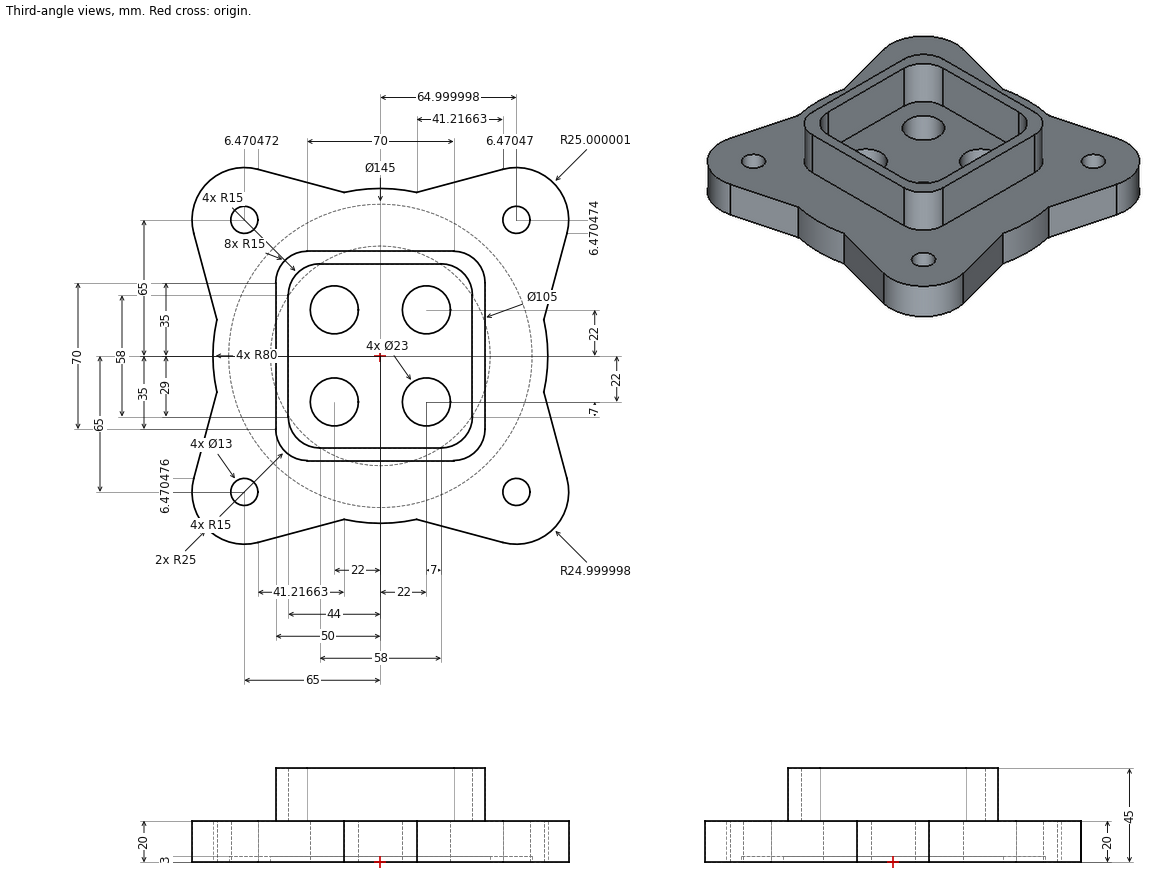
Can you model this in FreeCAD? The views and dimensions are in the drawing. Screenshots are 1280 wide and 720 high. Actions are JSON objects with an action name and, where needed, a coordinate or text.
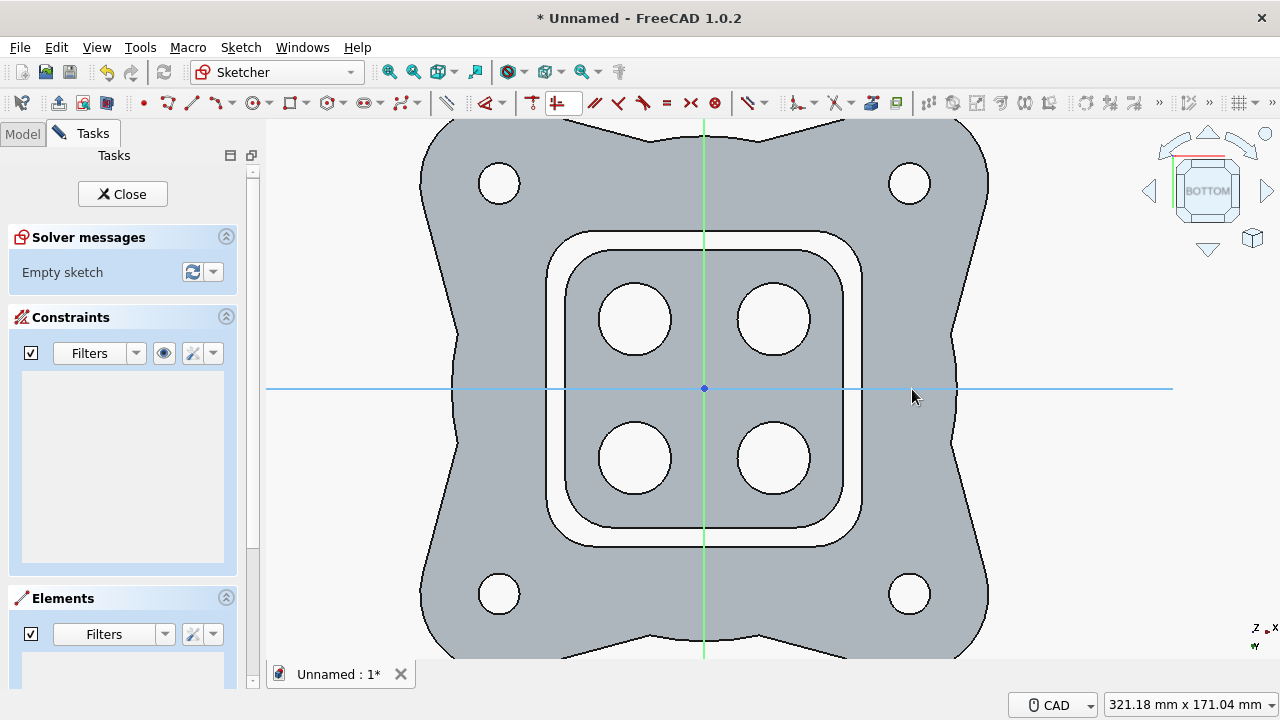
{"action": "key", "text": "g l"}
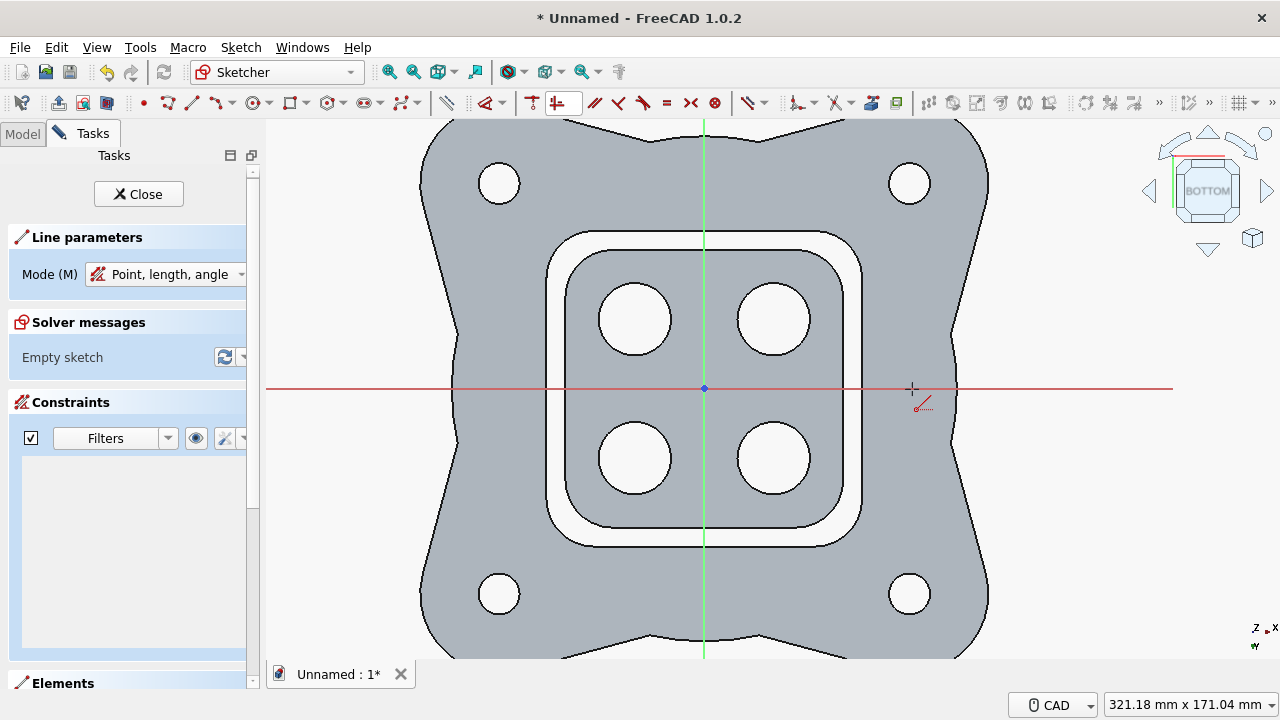
{"action": "left_click", "coordinate": [546, 499]}
{"action": "left_click", "coordinate": [546, 278]}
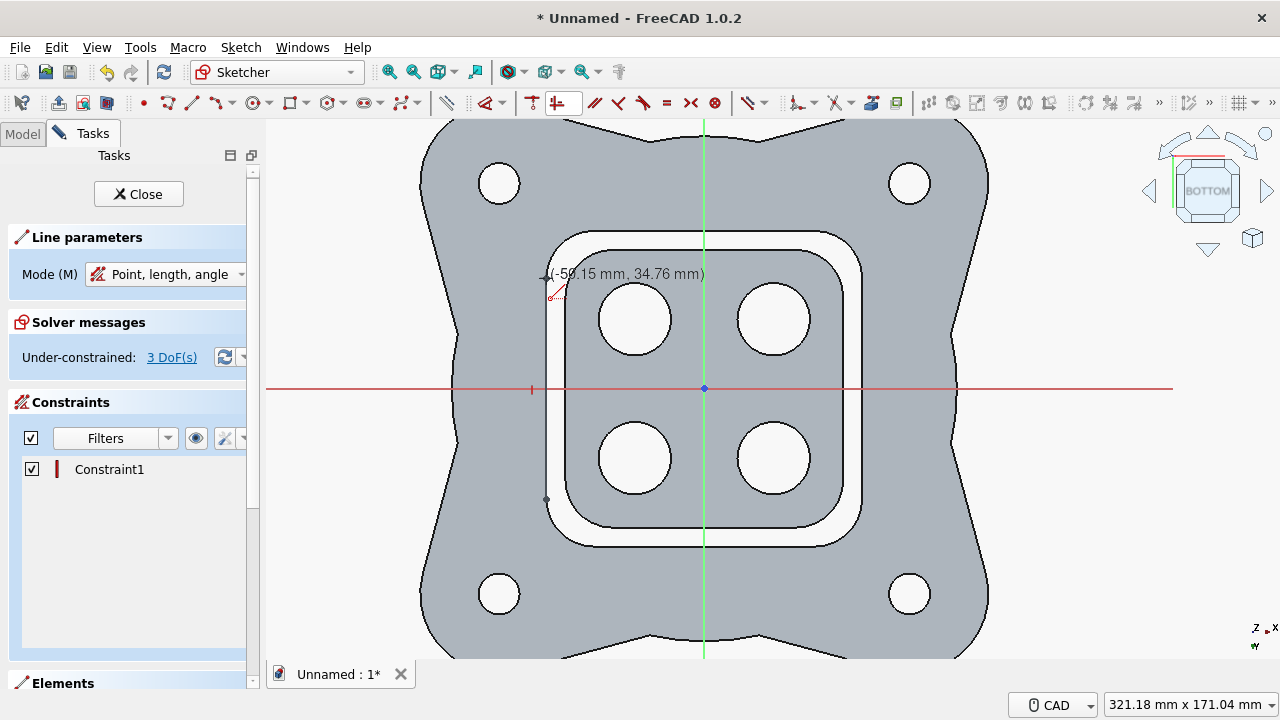
{"action": "left_click", "coordinate": [594, 231]}
{"action": "left_click", "coordinate": [815, 231]}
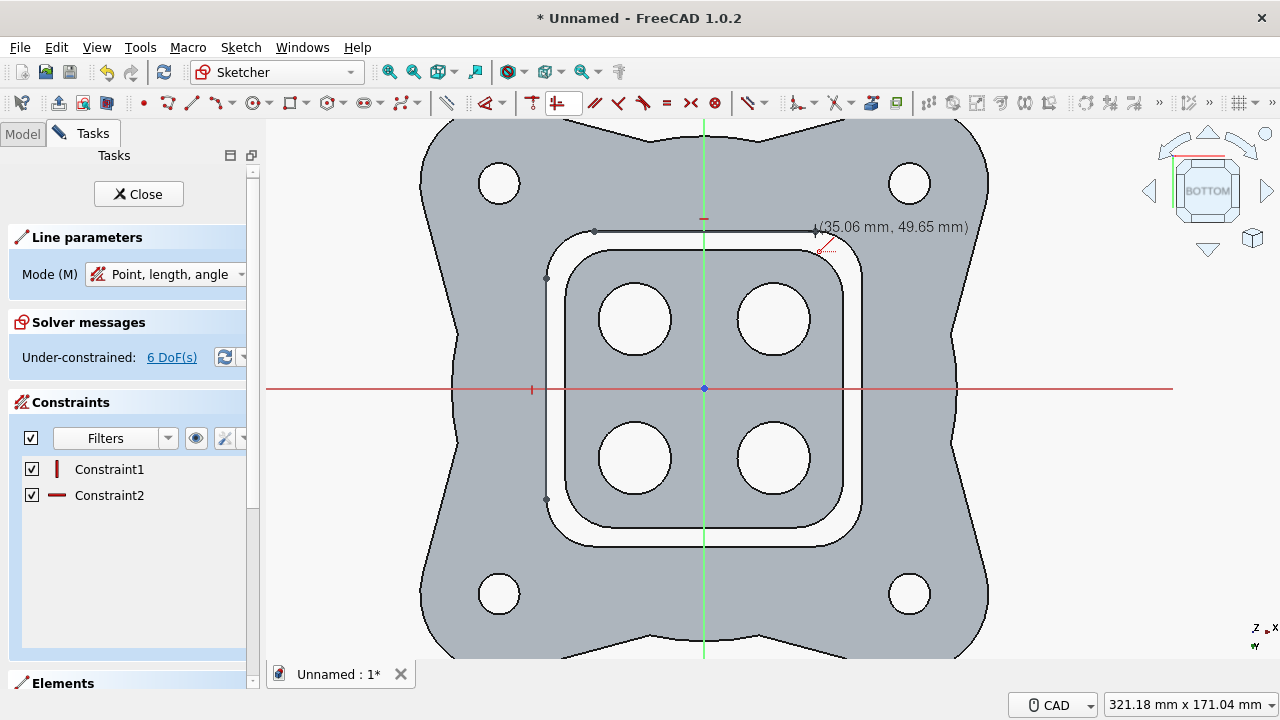
{"action": "left_click", "coordinate": [862, 278]}
{"action": "left_click", "coordinate": [862, 499]}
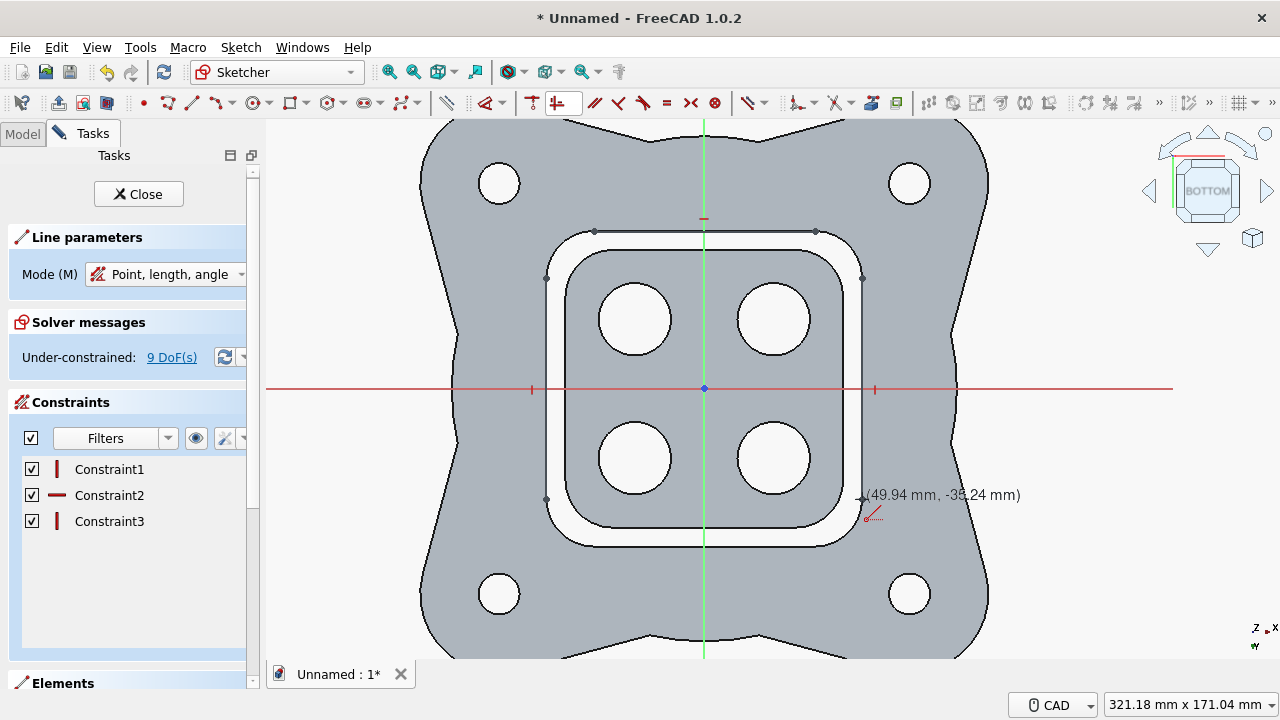
{"action": "left_click", "coordinate": [815, 547]}
{"action": "left_click", "coordinate": [594, 547]}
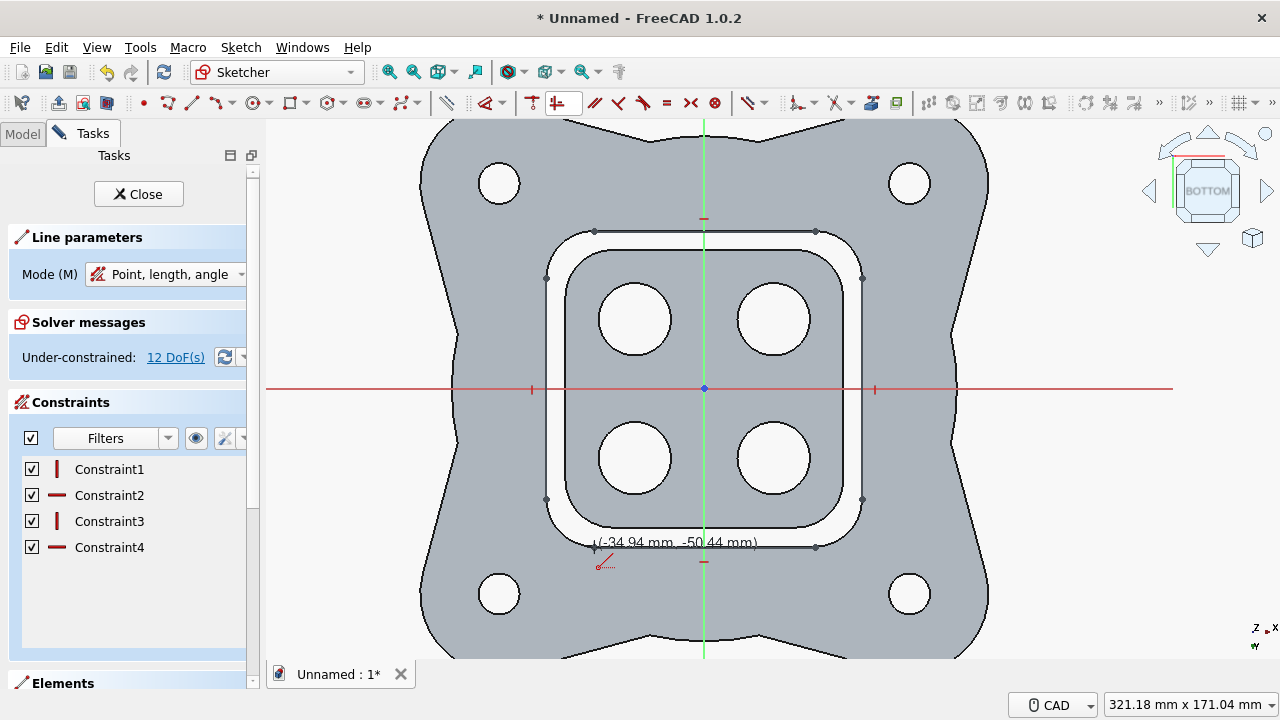
{"action": "key", "text": "g 3 a"}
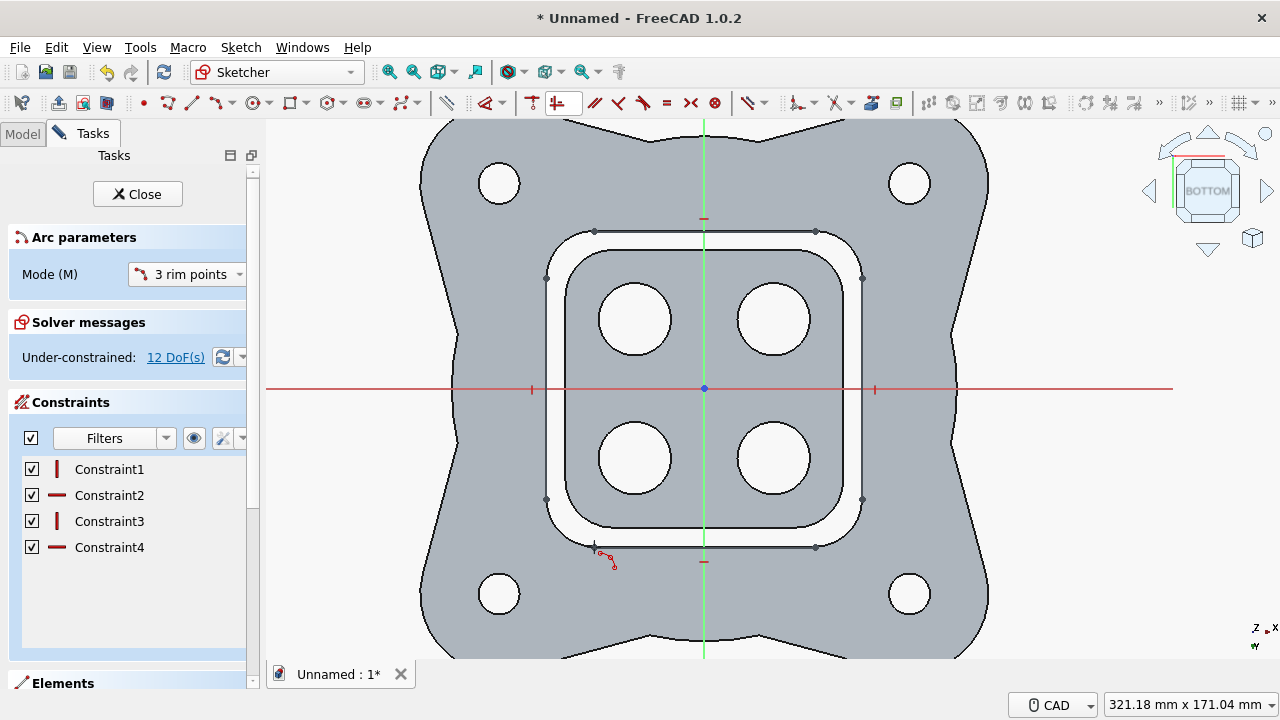
{"action": "left_click", "coordinate": [546, 279]}
{"action": "left_click", "coordinate": [594, 232]}
{"action": "left_click", "coordinate": [560, 245]}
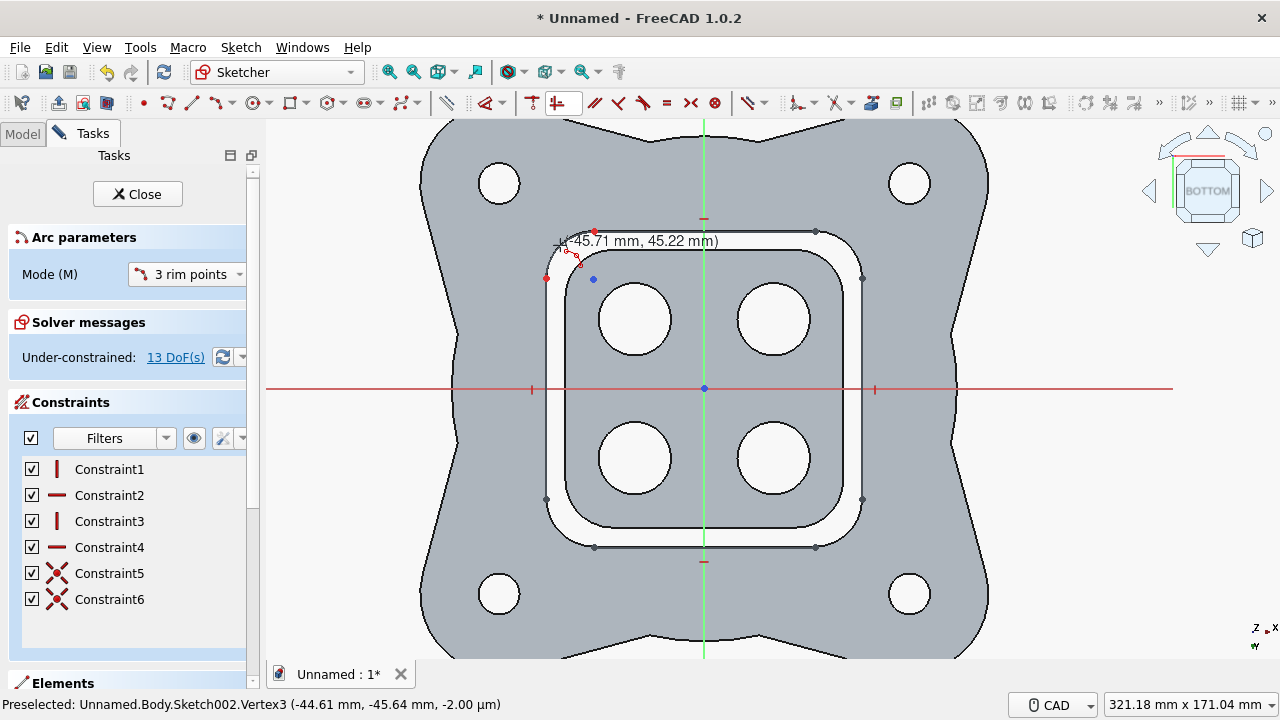
{"action": "left_click", "coordinate": [815, 232]}
{"action": "left_click", "coordinate": [862, 279]}
{"action": "left_click", "coordinate": [848, 245]}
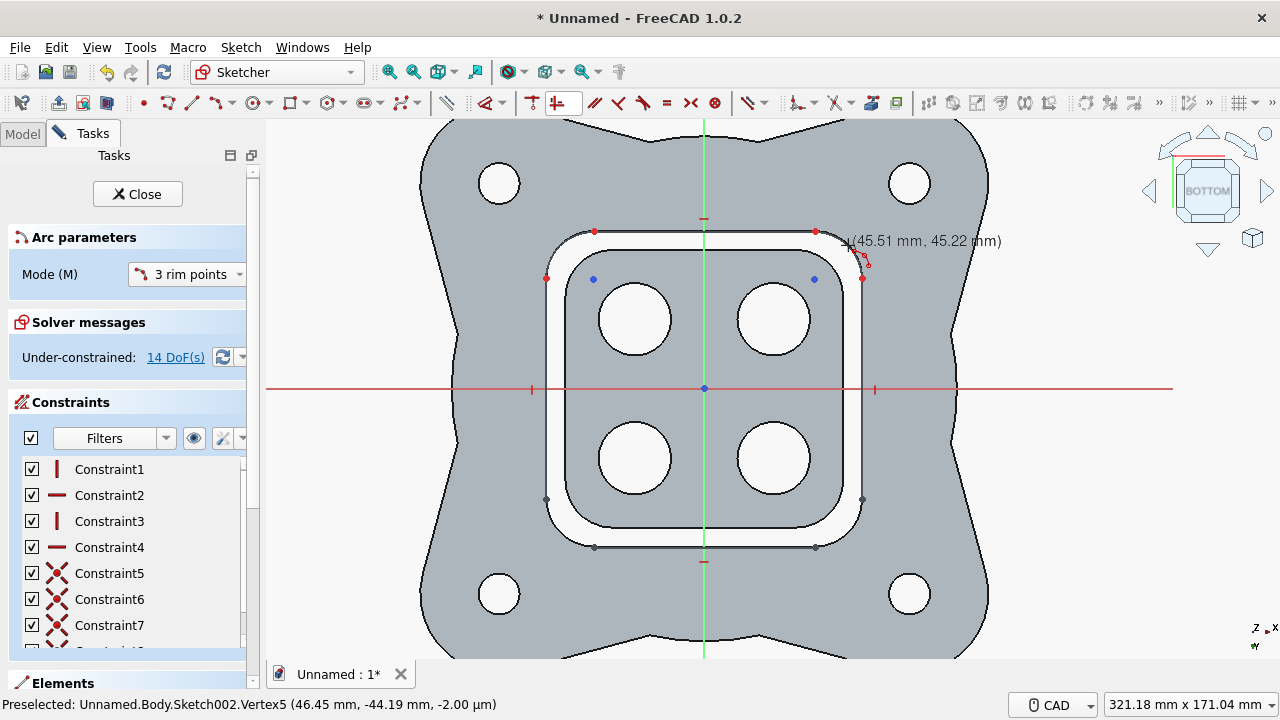
{"action": "left_click", "coordinate": [862, 500]}
{"action": "left_click", "coordinate": [815, 548]}
{"action": "left_click", "coordinate": [848, 533]}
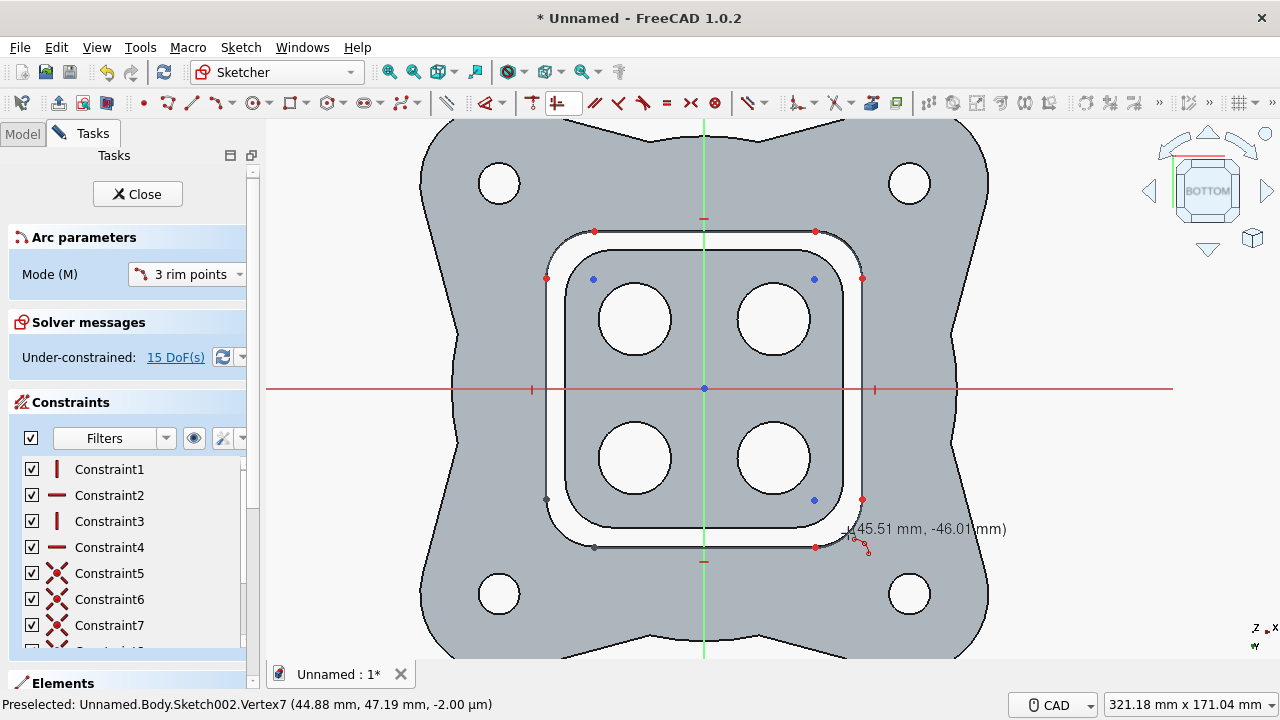
{"action": "left_click", "coordinate": [594, 548]}
{"action": "left_click", "coordinate": [546, 500]}
{"action": "left_click", "coordinate": [560, 533]}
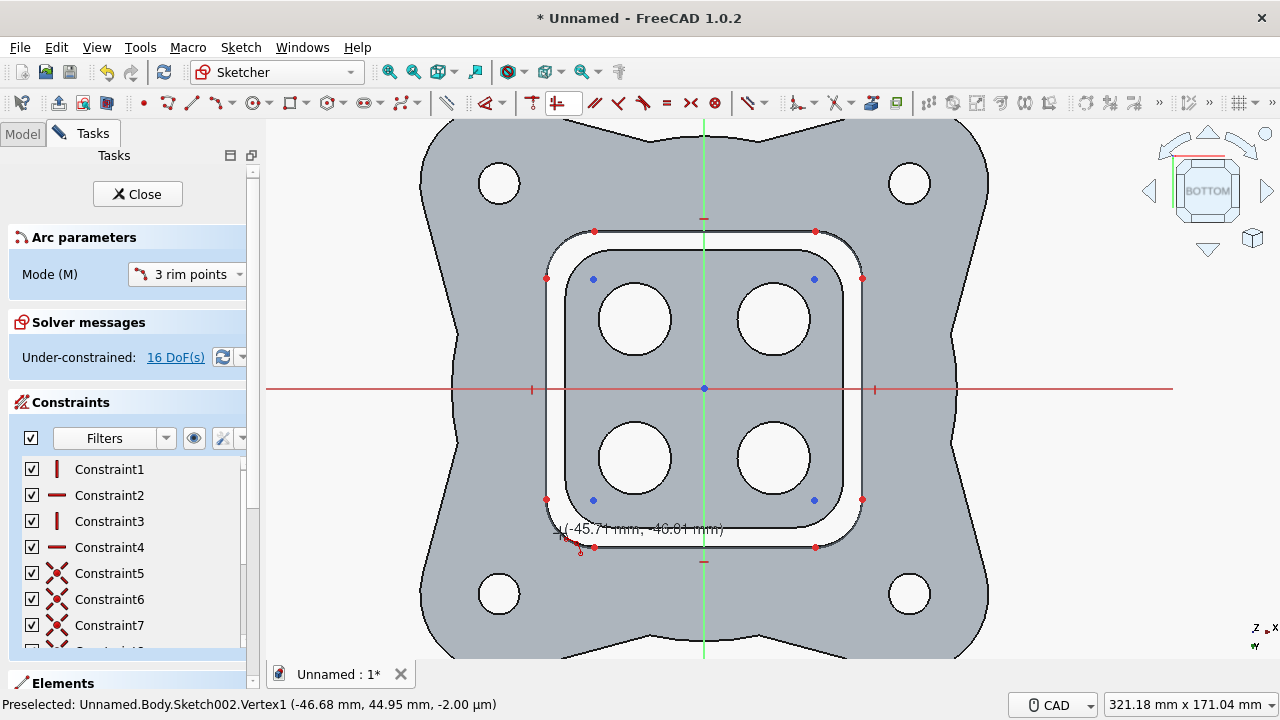
{"action": "left_click", "coordinate": [192, 104]}